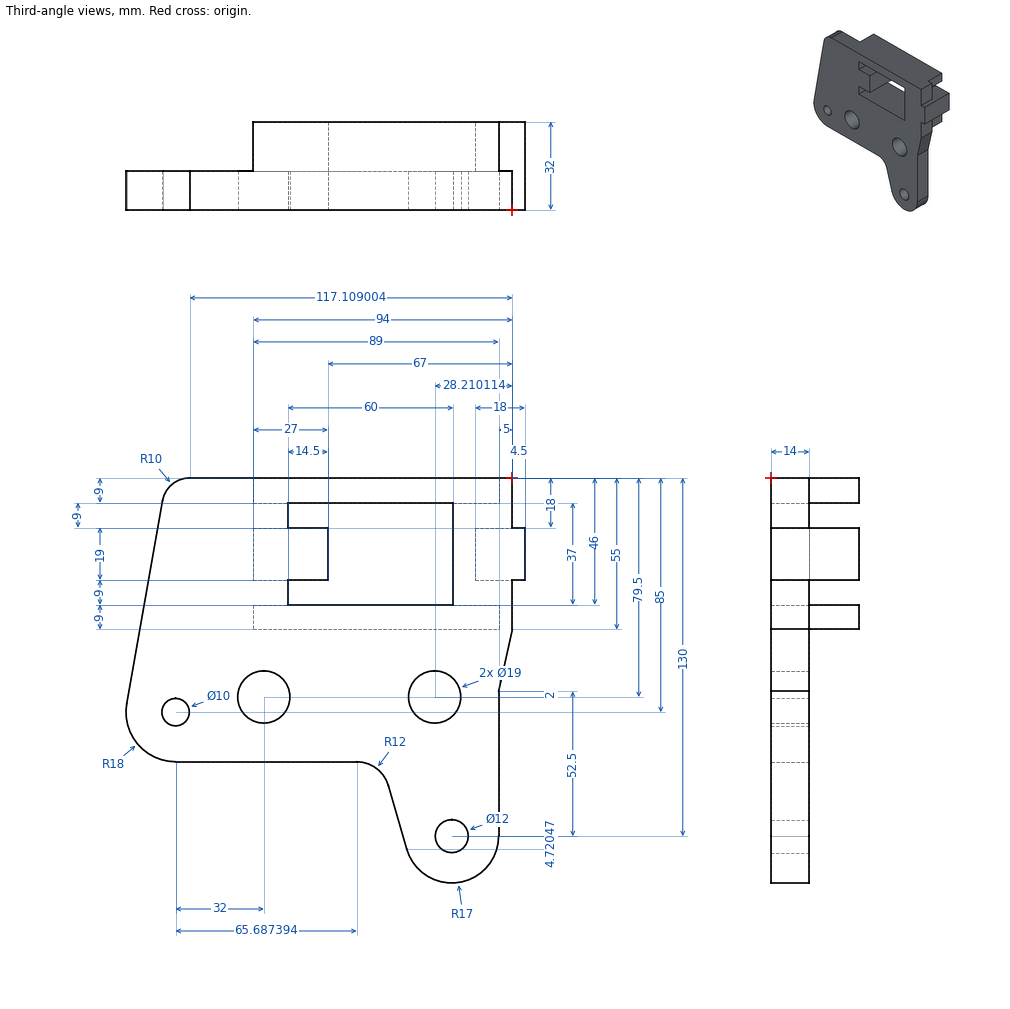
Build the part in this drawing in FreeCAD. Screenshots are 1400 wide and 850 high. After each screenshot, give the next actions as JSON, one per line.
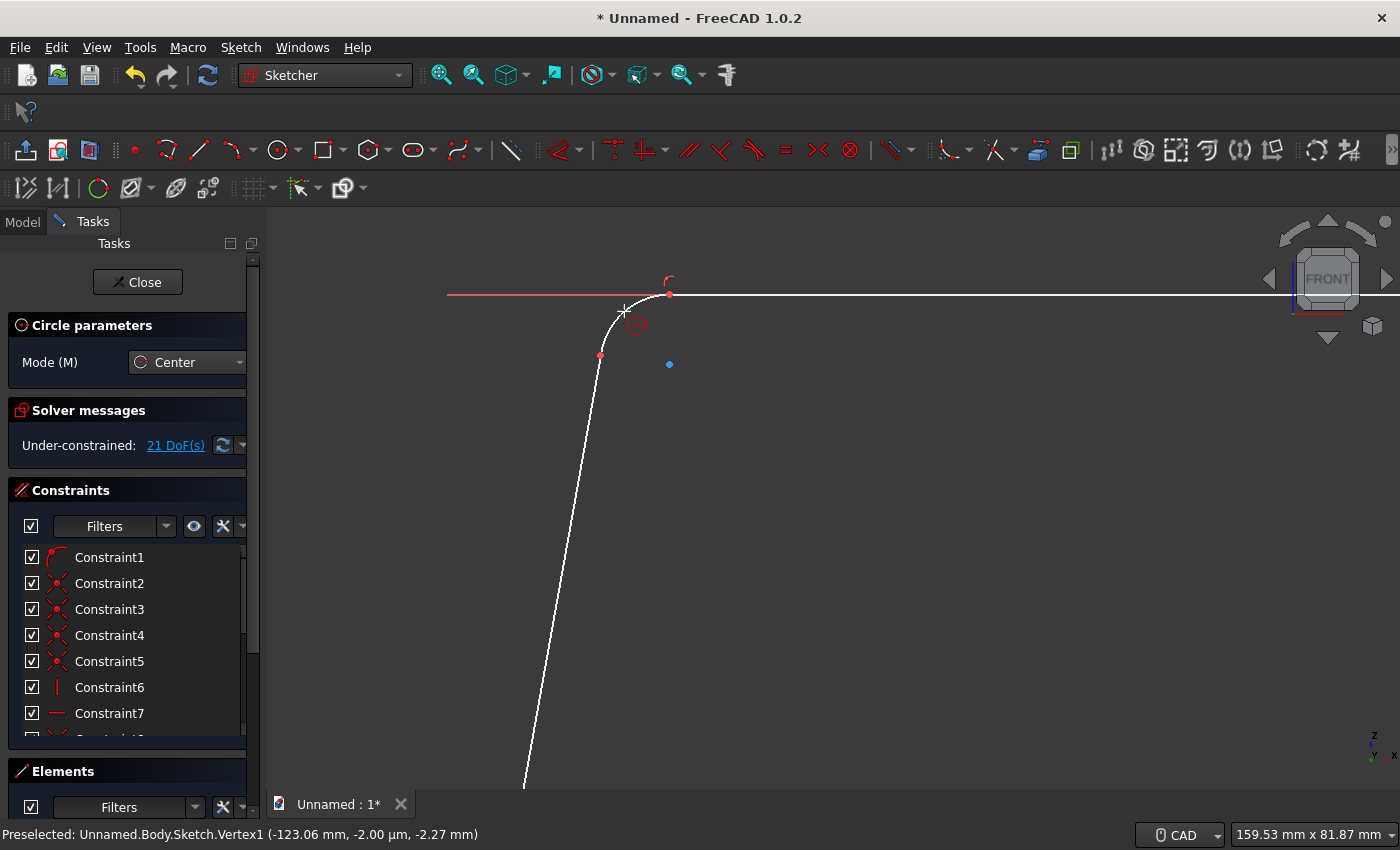
{"action": "scroll", "coordinate": [625, 313], "scroll_direction": "down", "scroll_amount": 5}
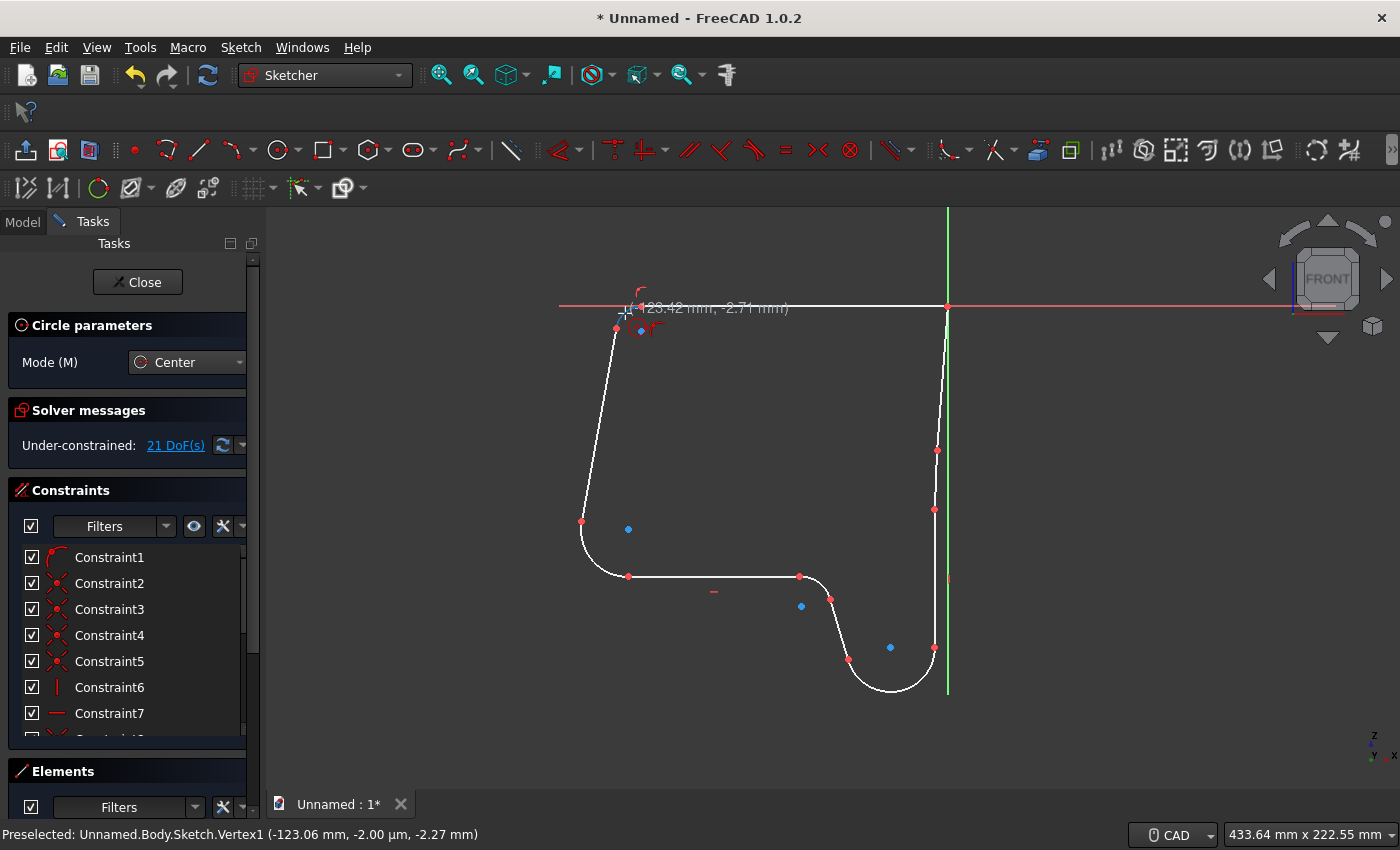
{"action": "left_click", "coordinate": [874, 514]}
{"action": "left_click", "coordinate": [892, 497]}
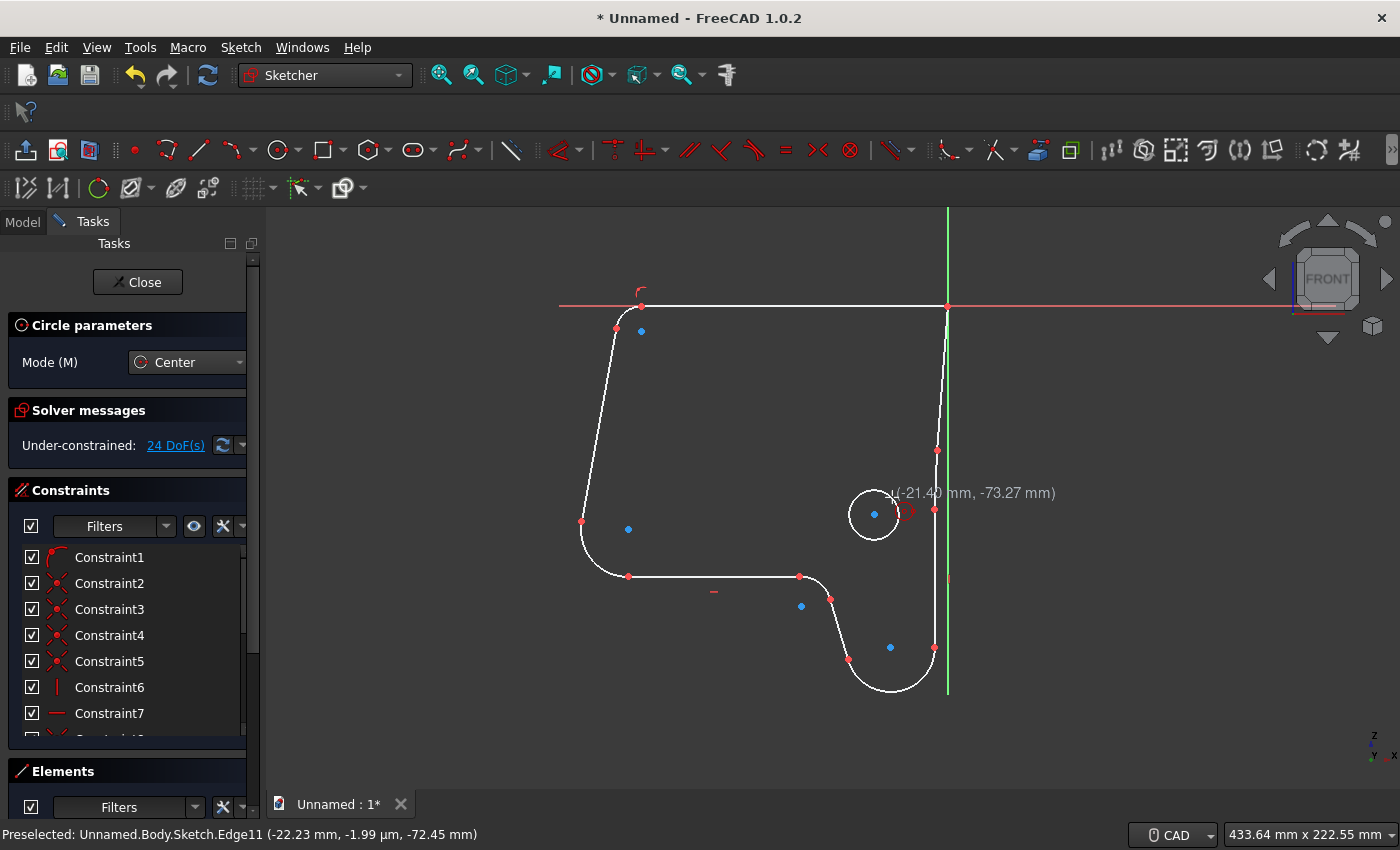
{"action": "left_click", "coordinate": [712, 514]}
{"action": "left_click", "coordinate": [730, 497]}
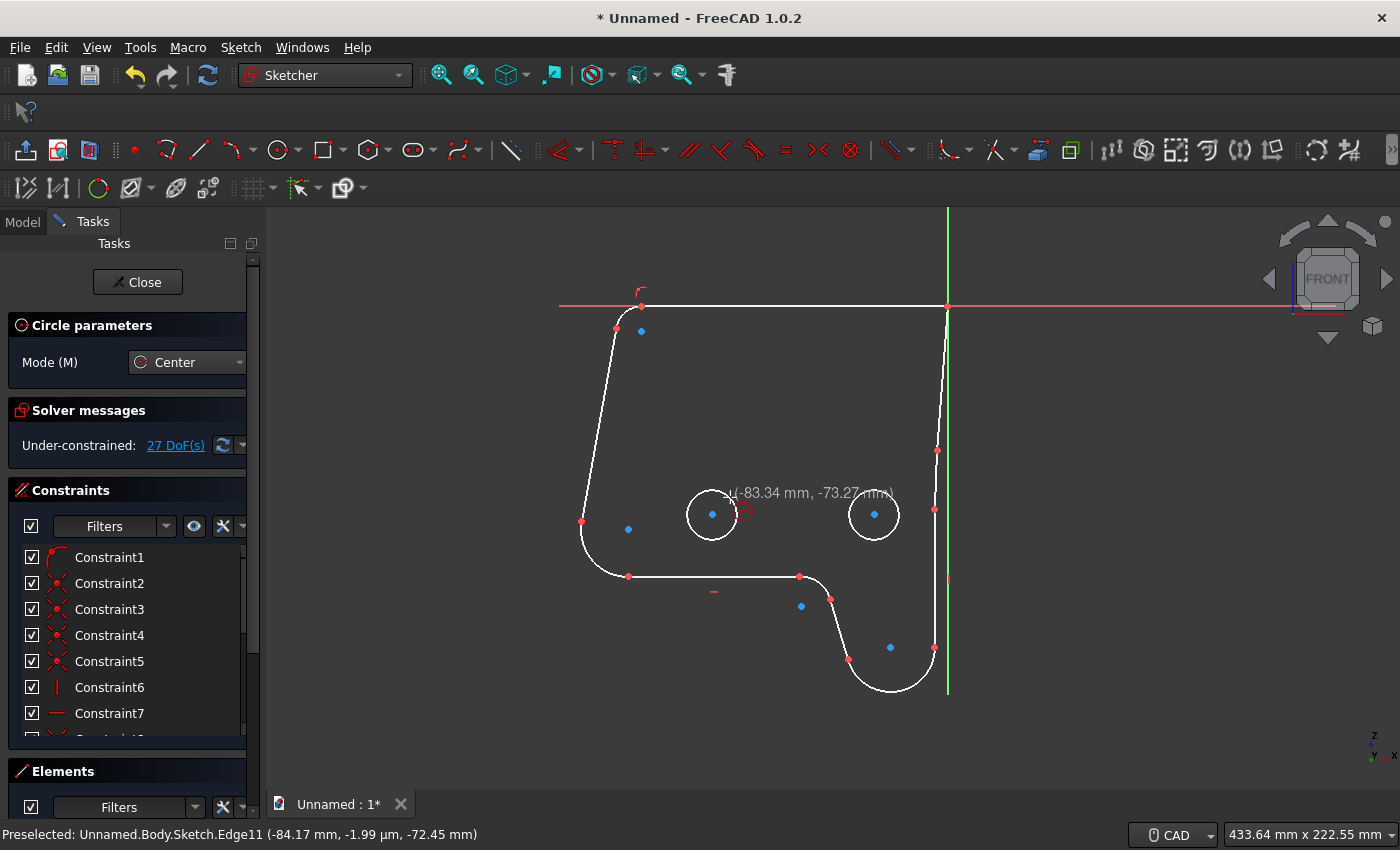
{"action": "scroll", "coordinate": [628, 529], "scroll_direction": "up", "scroll_amount": 3}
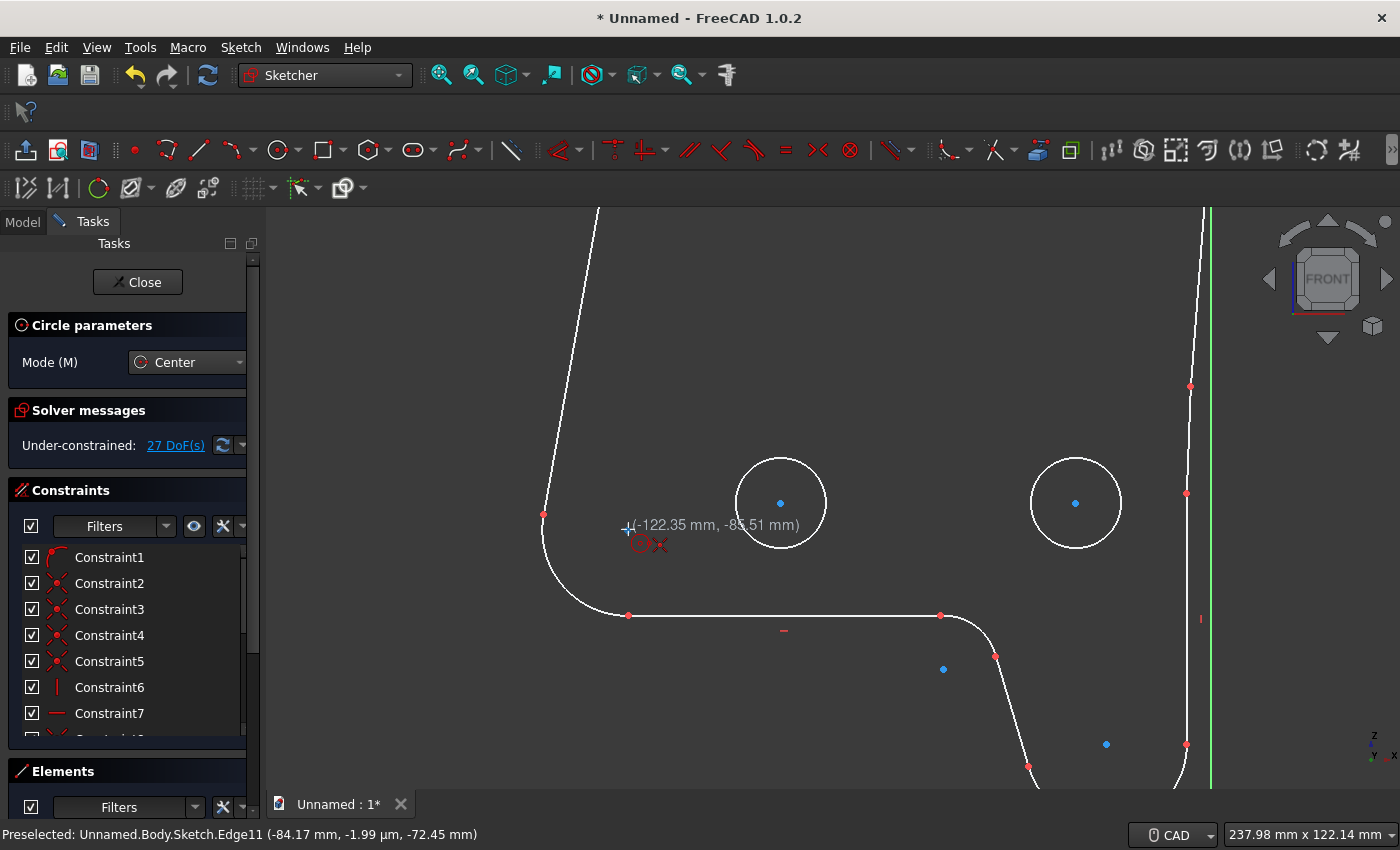
{"action": "left_click", "coordinate": [628, 528]}
{"action": "left_click", "coordinate": [645, 511]}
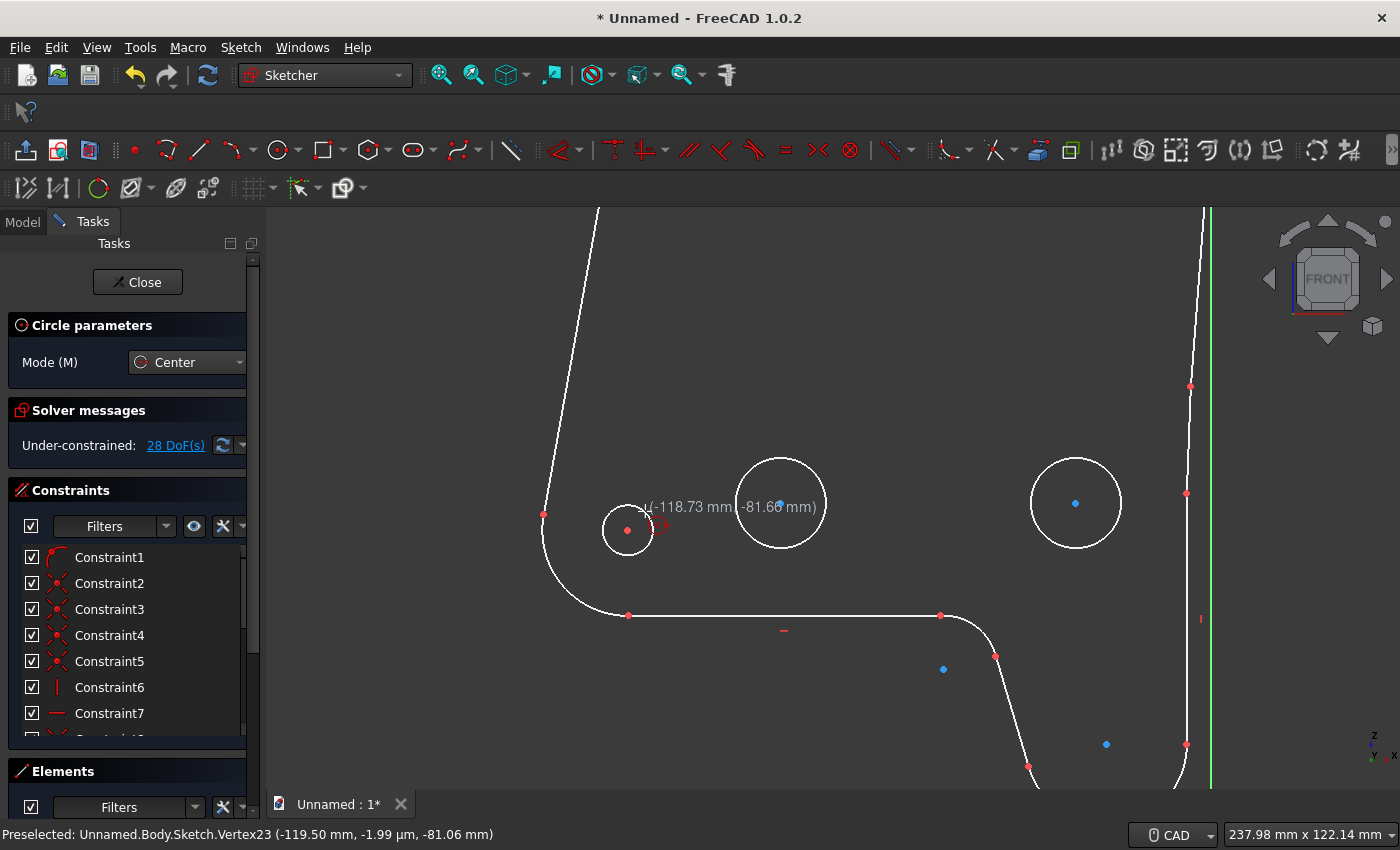
{"action": "left_click", "coordinate": [1106, 742]}
{"action": "left_click", "coordinate": [1126, 722]}
{"action": "key", "text": "Escape"}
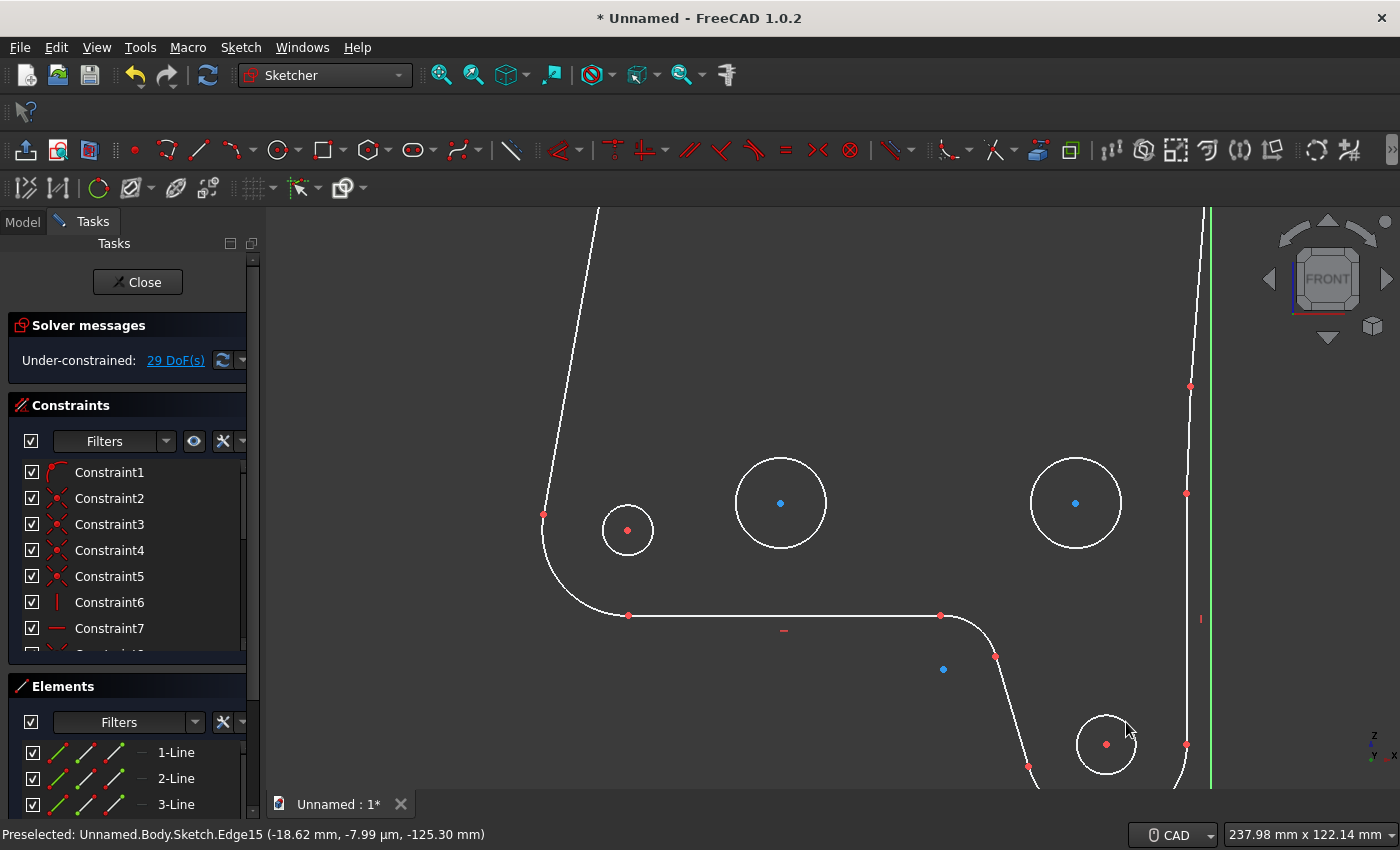
{"action": "scroll", "coordinate": [627, 529], "scroll_direction": "down", "scroll_amount": 3}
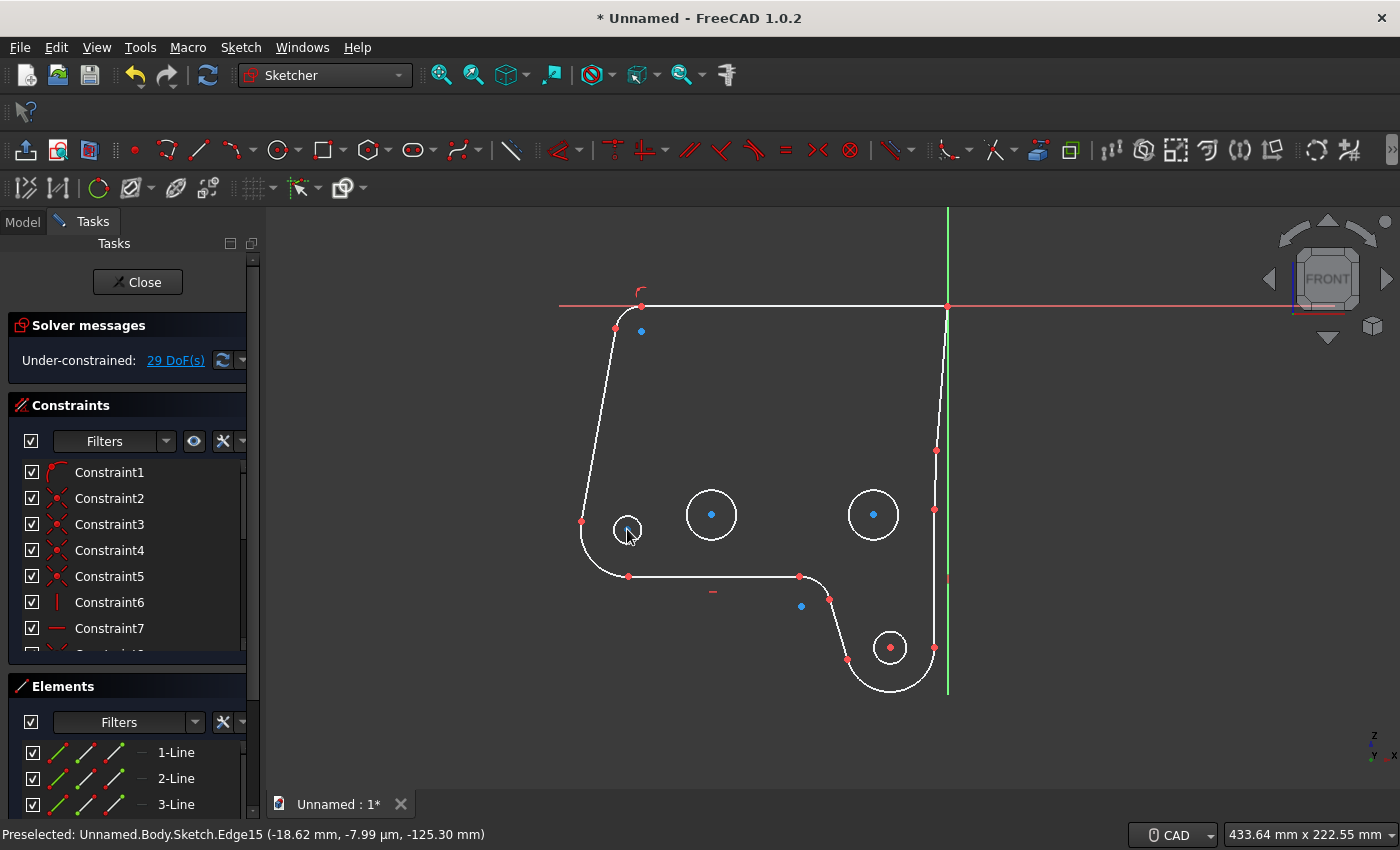
{"action": "left_click", "coordinate": [733, 306]}